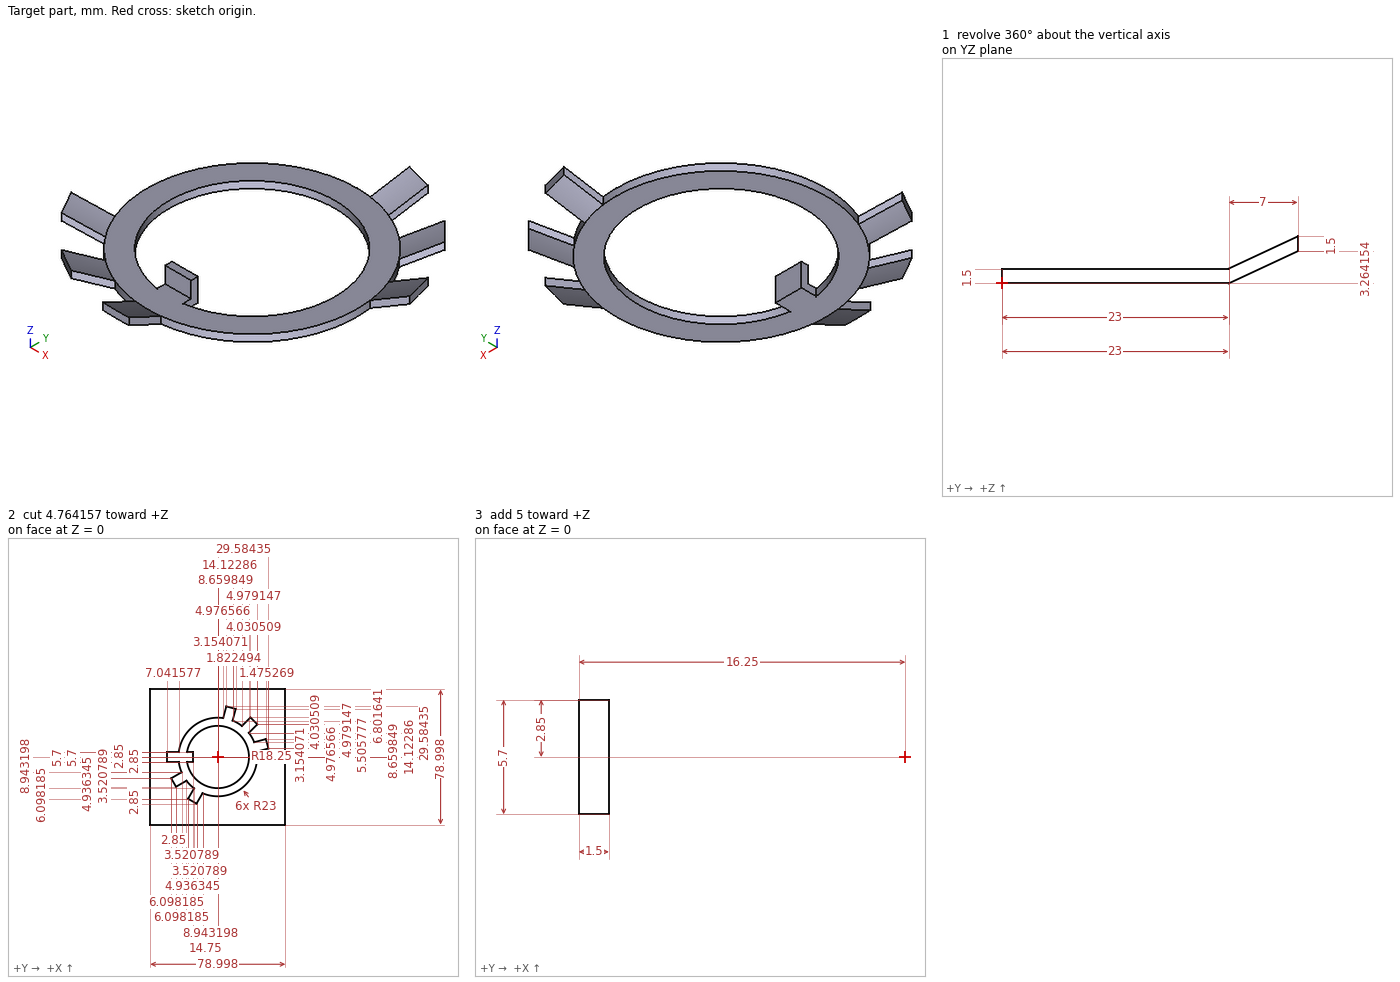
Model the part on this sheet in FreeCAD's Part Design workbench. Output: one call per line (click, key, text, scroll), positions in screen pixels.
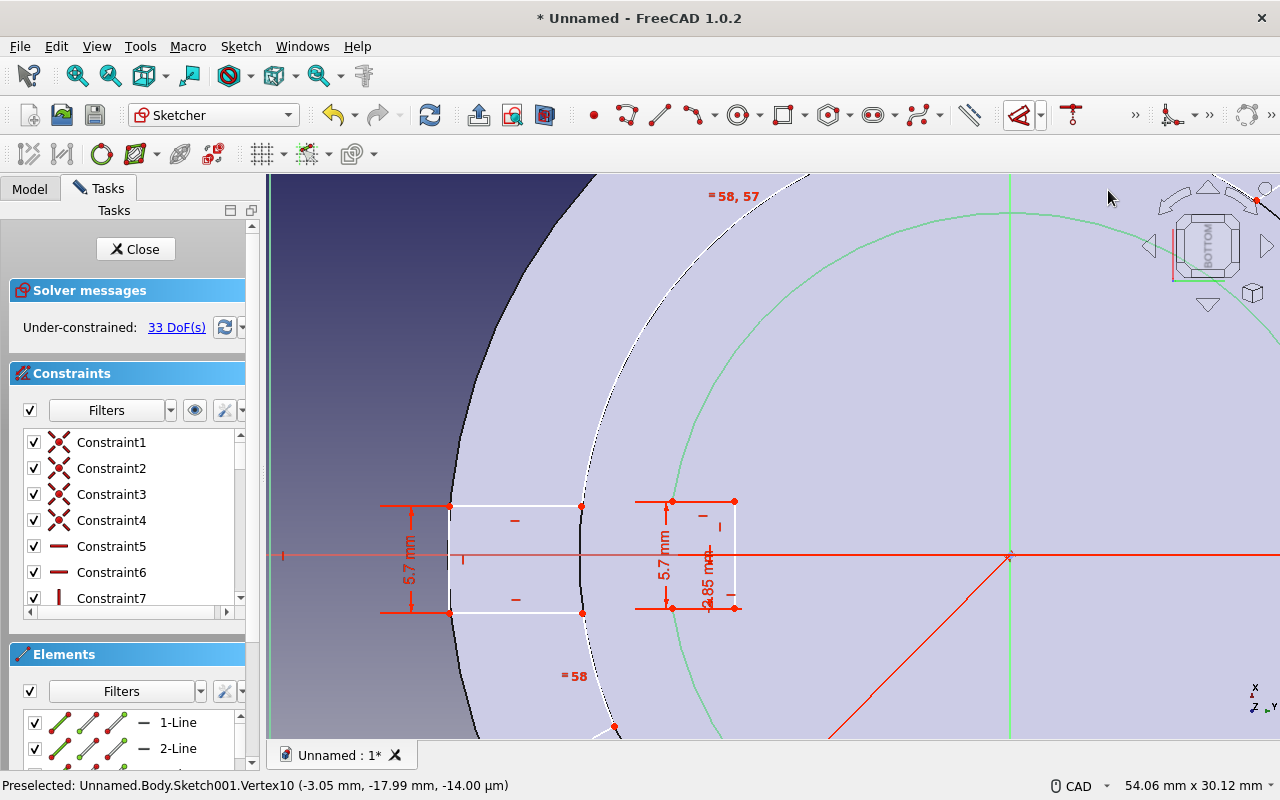
click(582, 506)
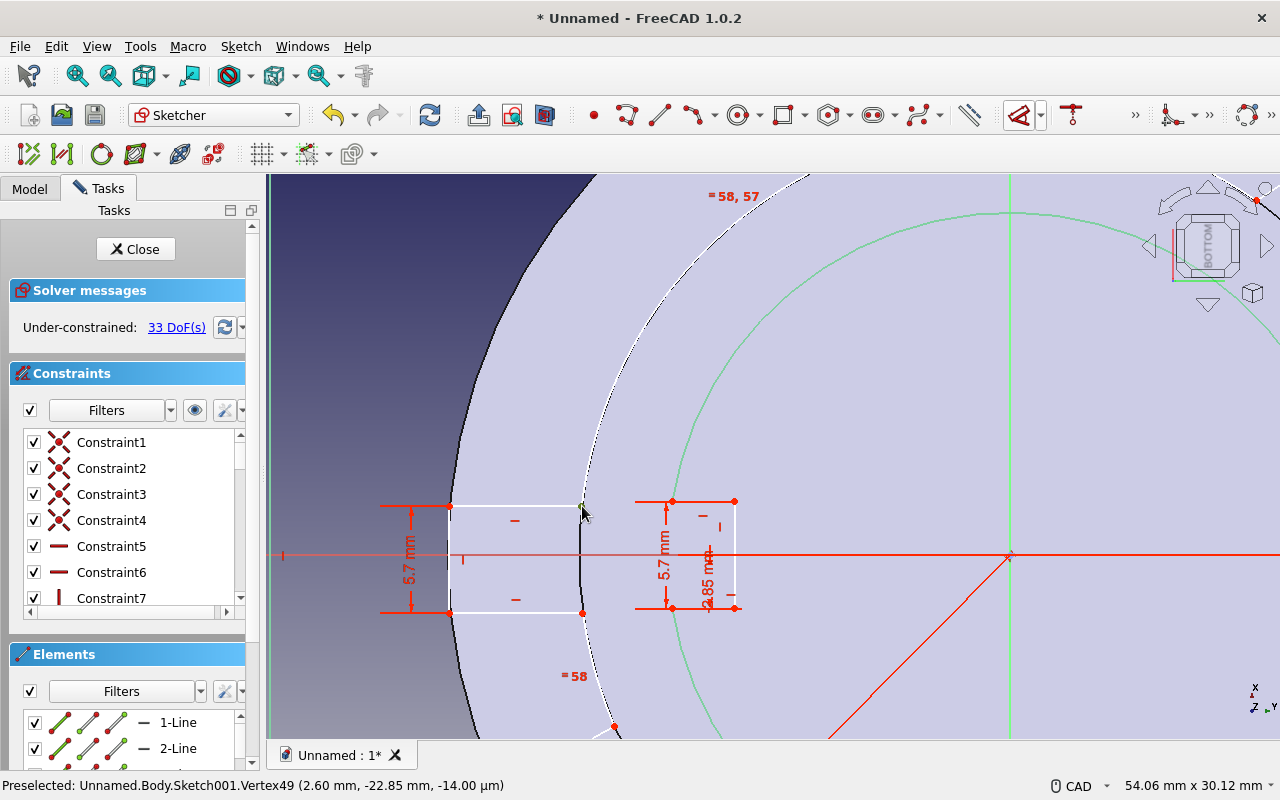
key(i)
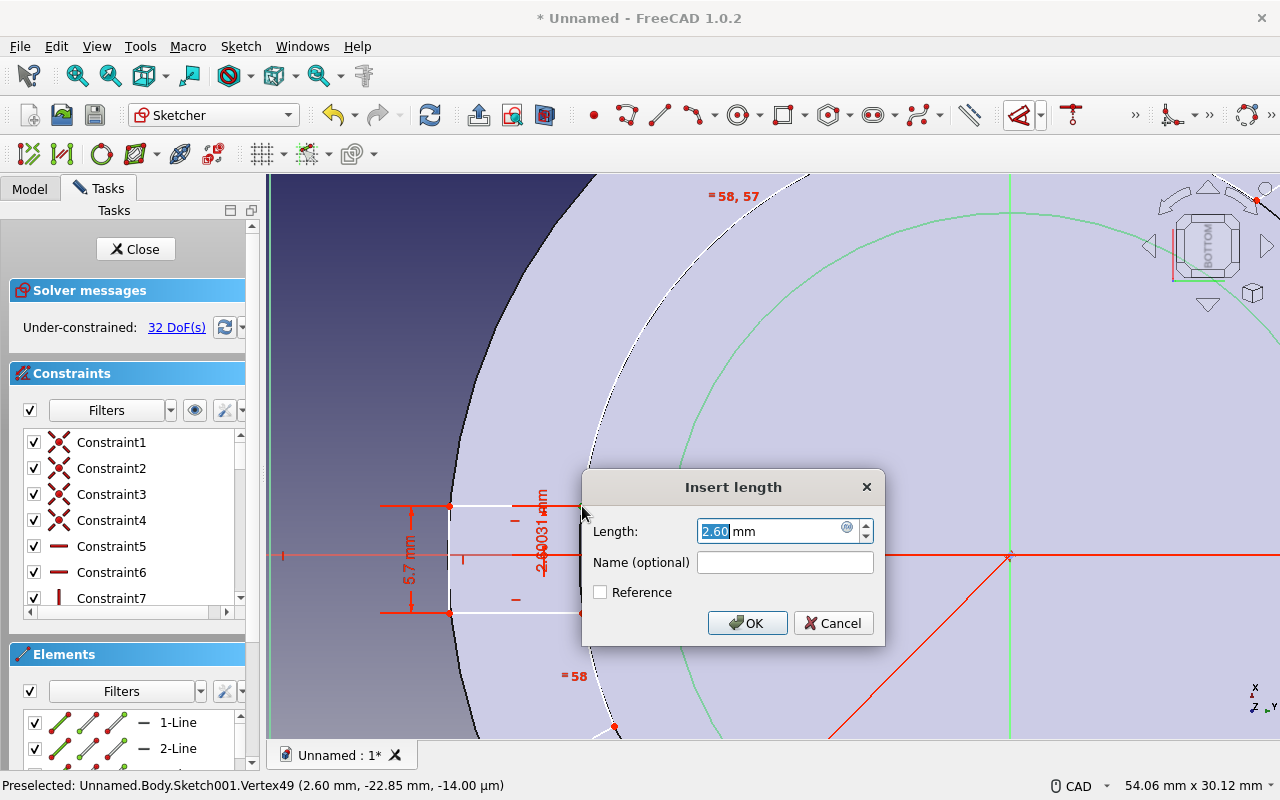
text(2.85)
key(Return)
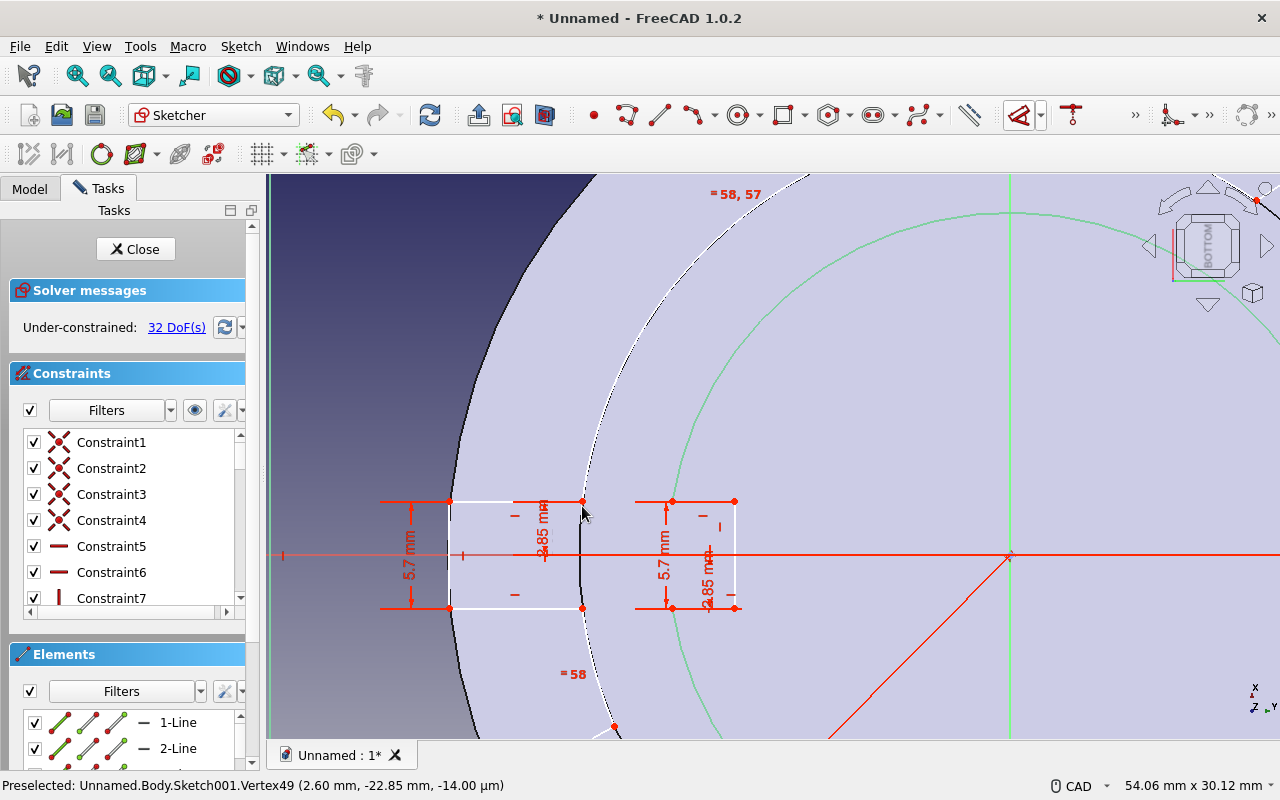
scroll(604, 424, down, 7)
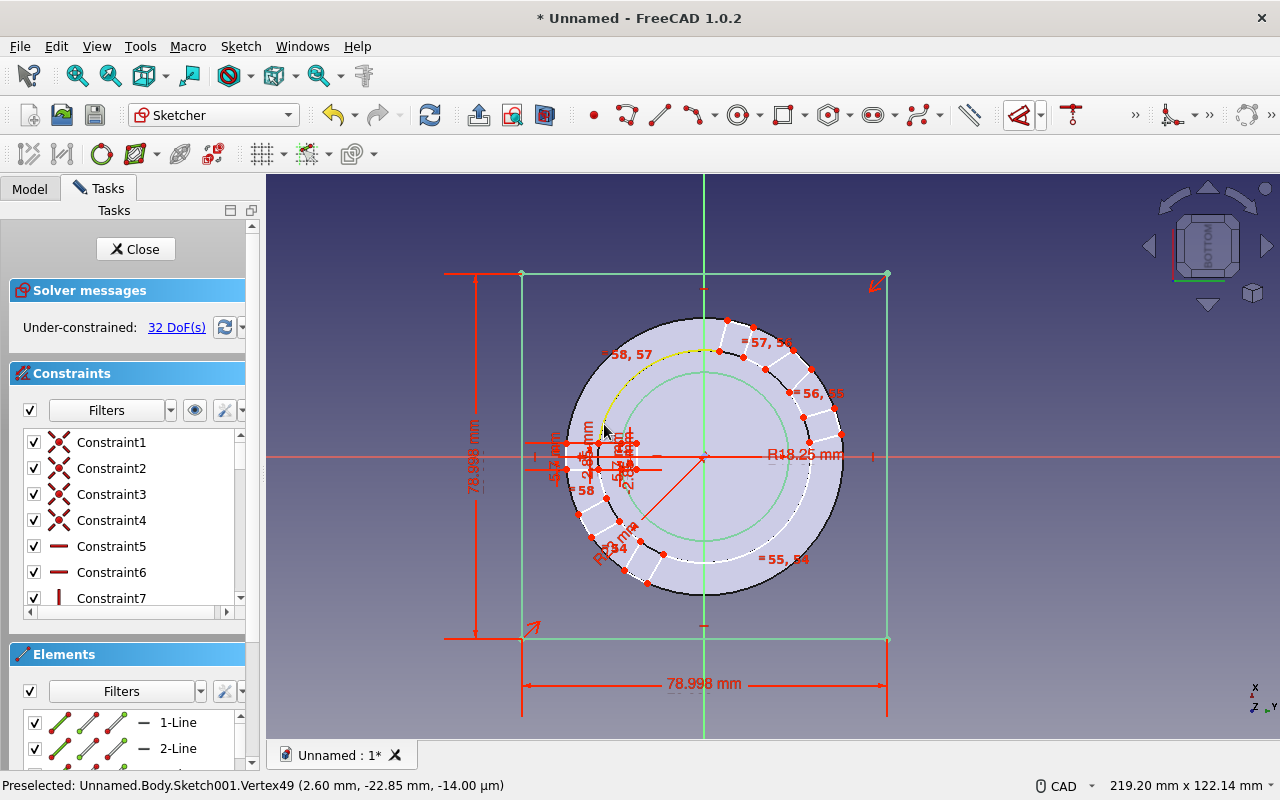
scroll(582, 522, up, 6)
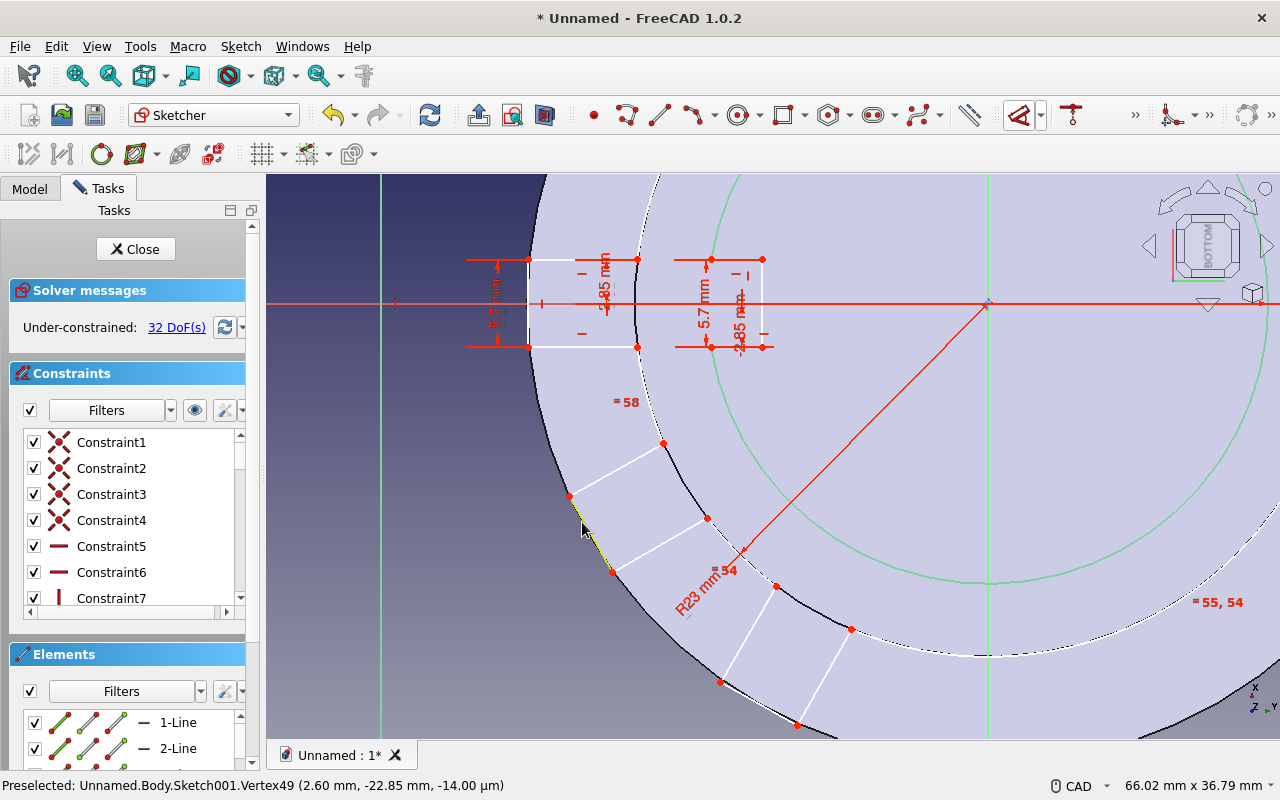
click(582, 519)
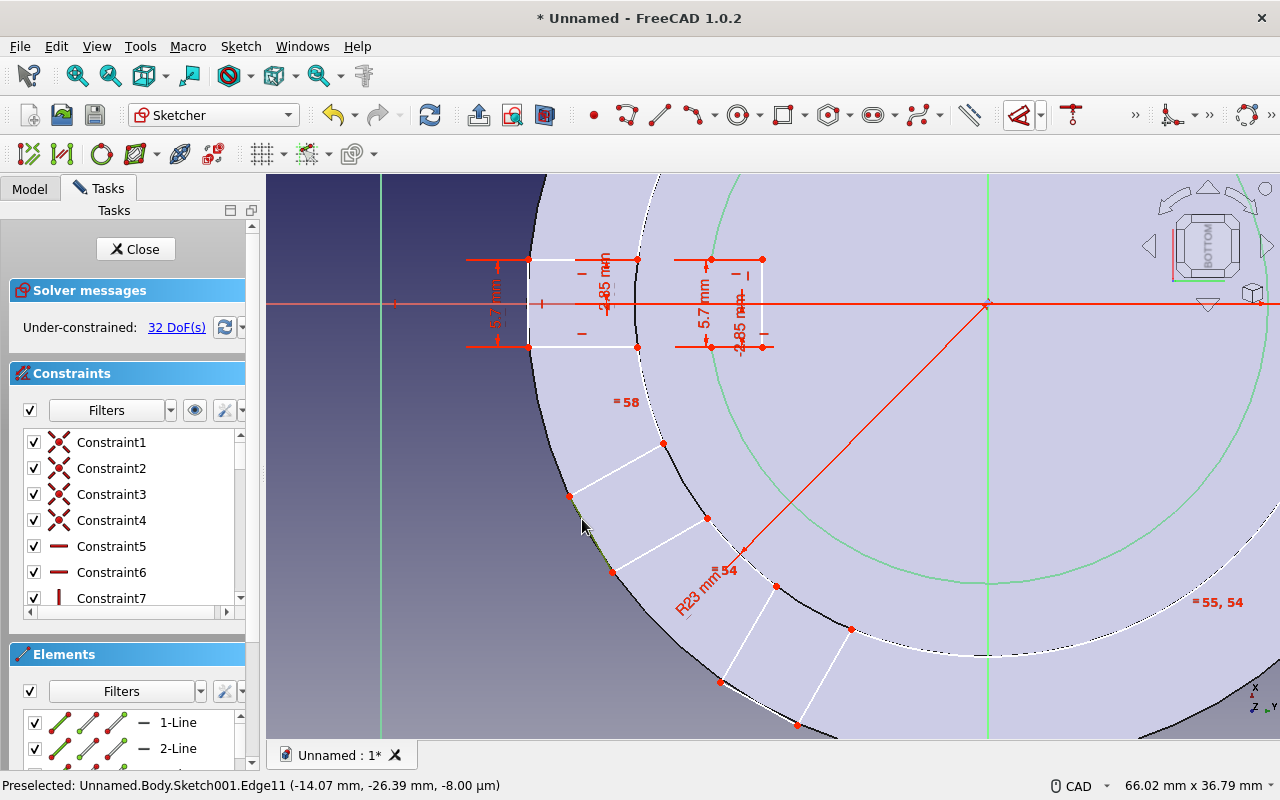
click(1040, 116)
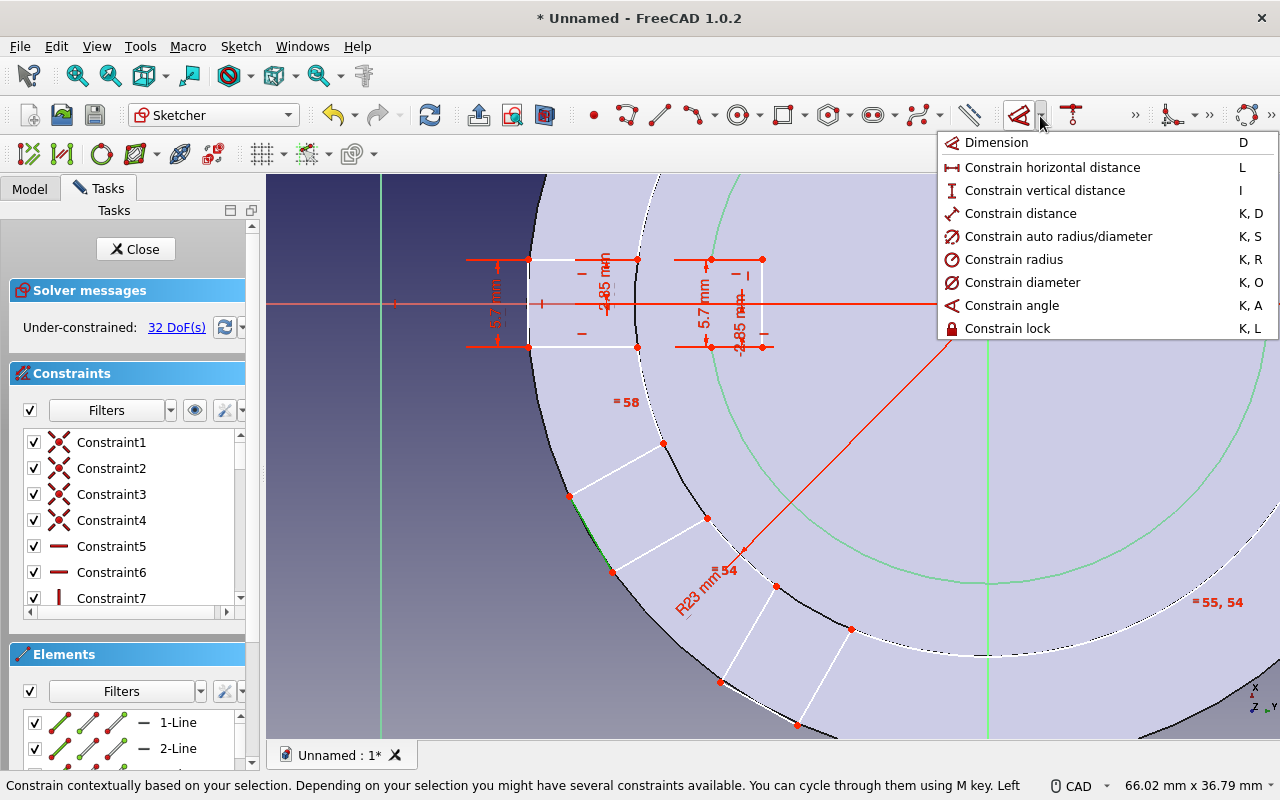
click(1108, 168)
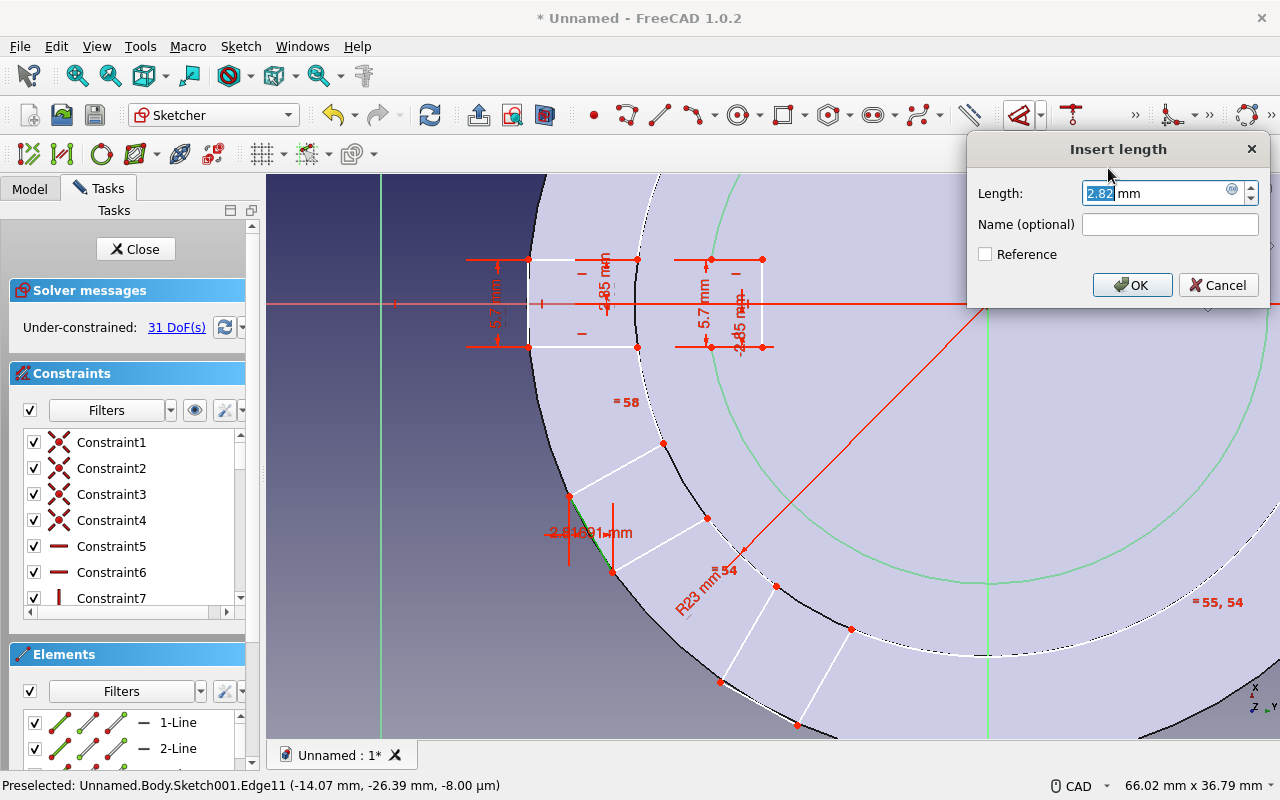
text(2.85)
key(Return)